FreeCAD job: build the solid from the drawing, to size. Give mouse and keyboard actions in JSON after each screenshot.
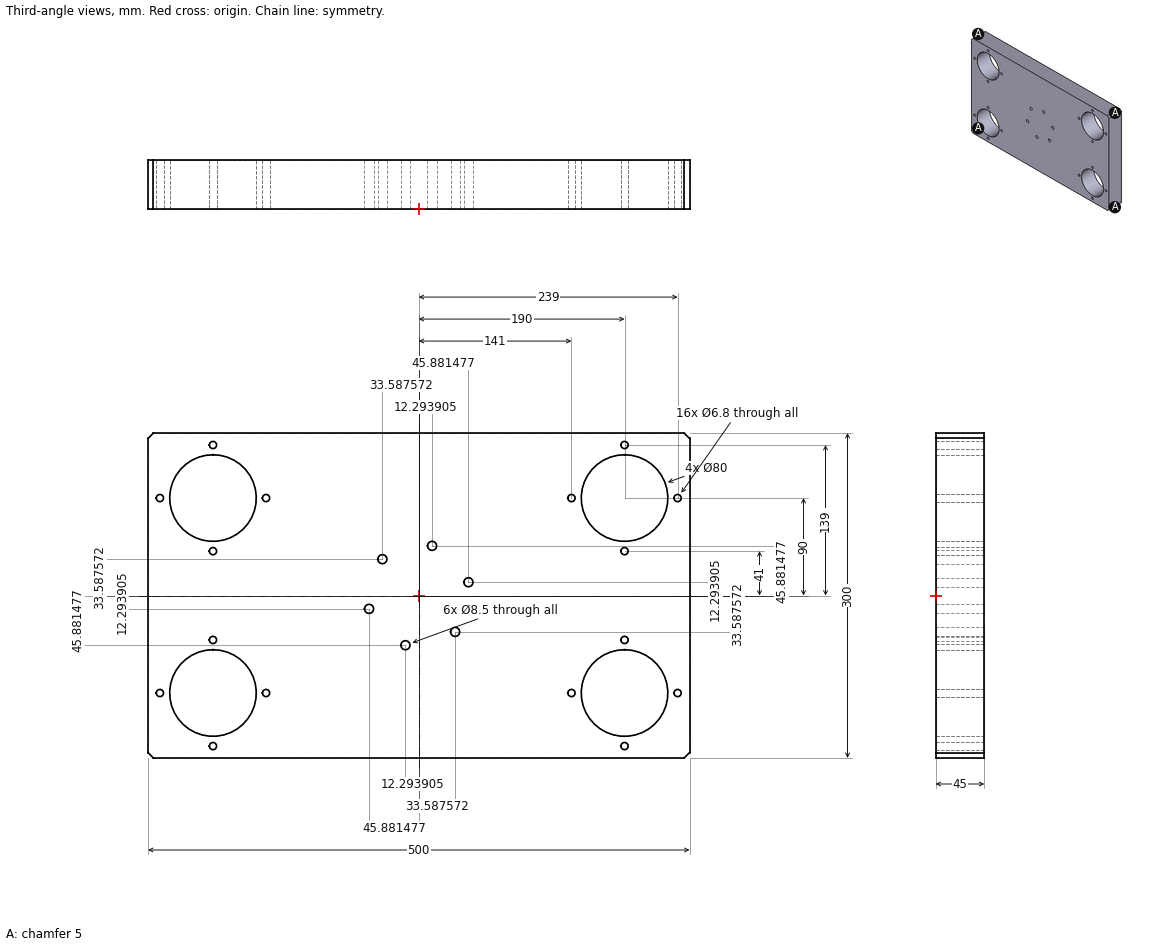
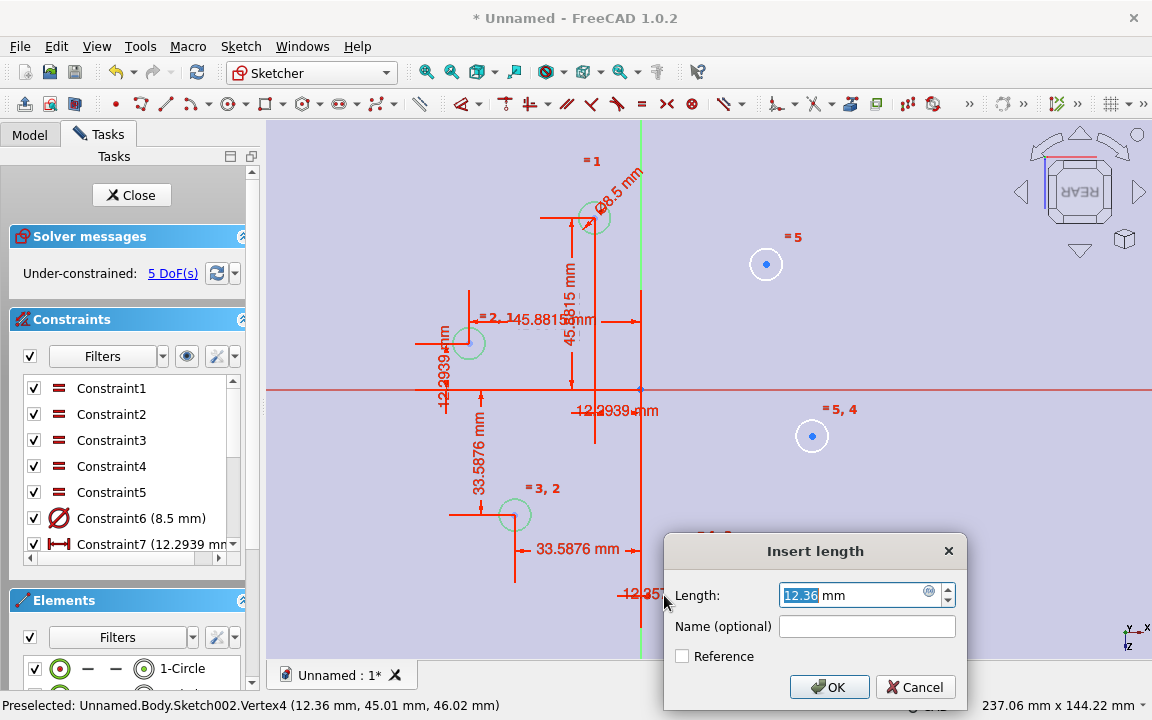
{"action": "type", "text": "12.293905"}
{"action": "key", "text": "Return"}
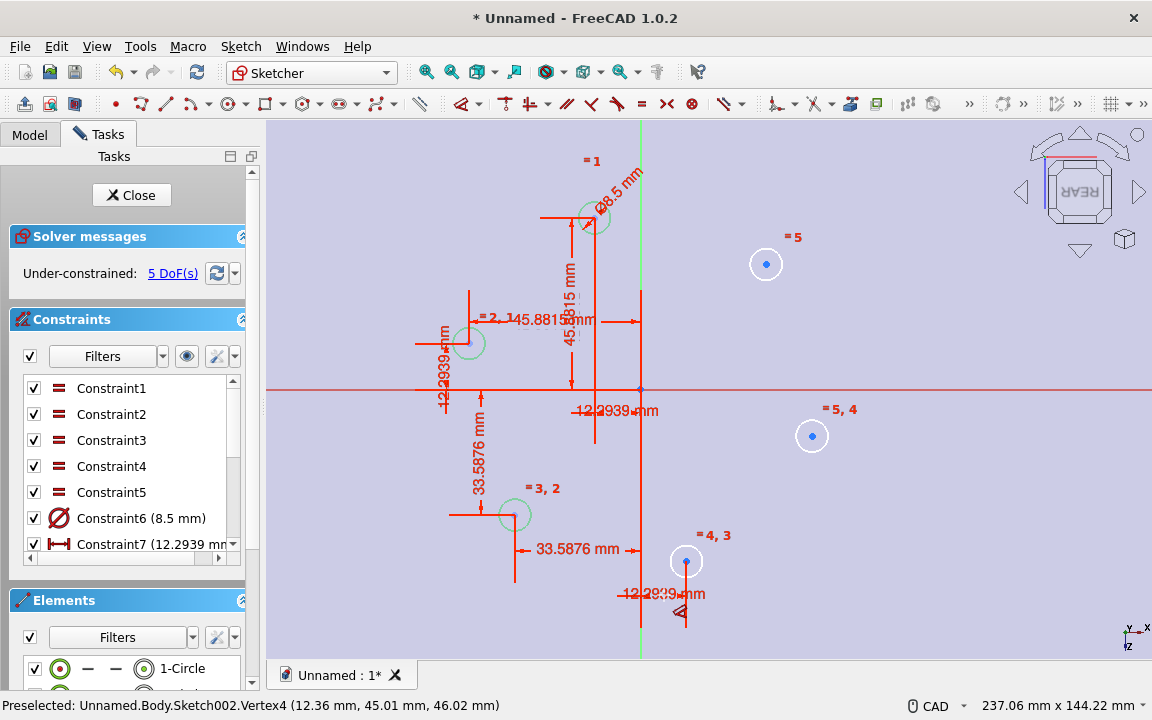
{"action": "left_click", "coordinate": [686, 561]}
{"action": "left_click", "coordinate": [720, 475]}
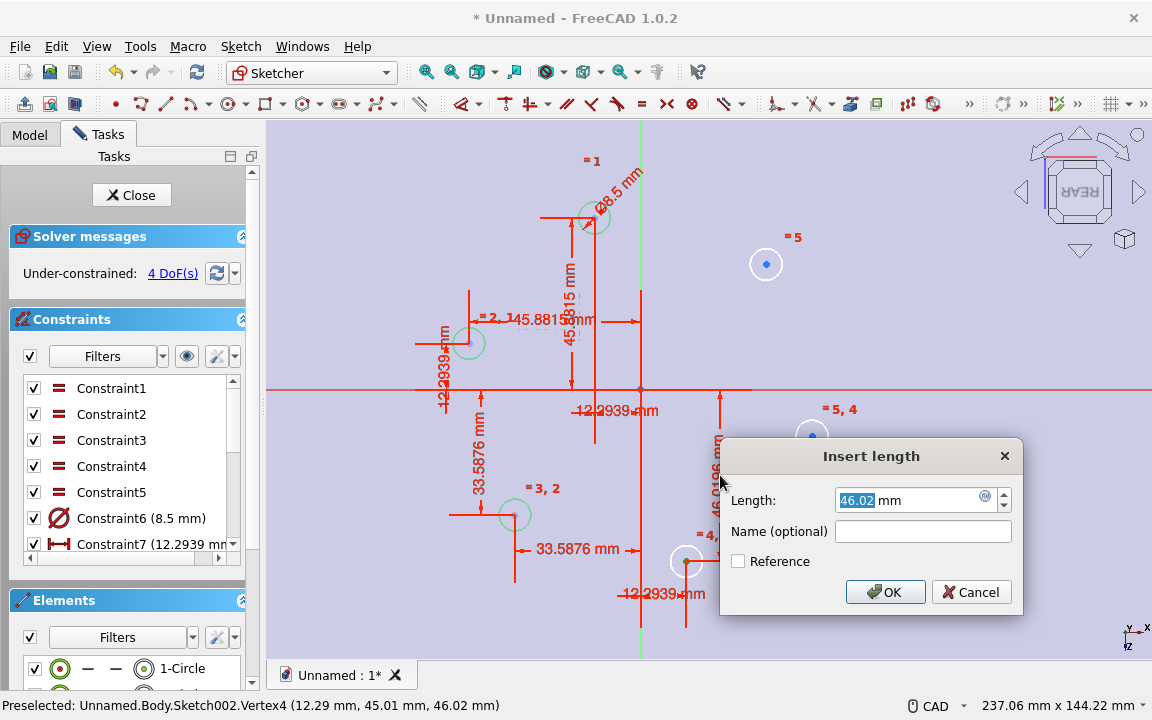
{"action": "type", "text": "45.881477"}
{"action": "key", "text": "Return"}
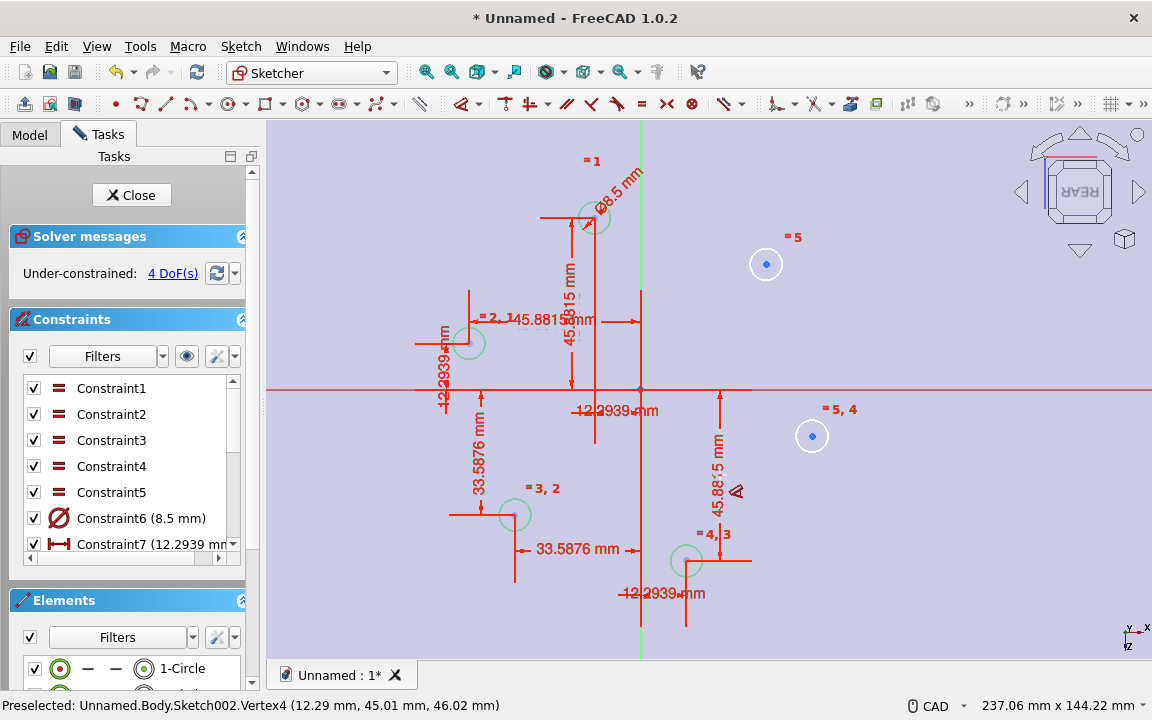
{"action": "left_click", "coordinate": [812, 436]}
{"action": "left_click", "coordinate": [726, 355]}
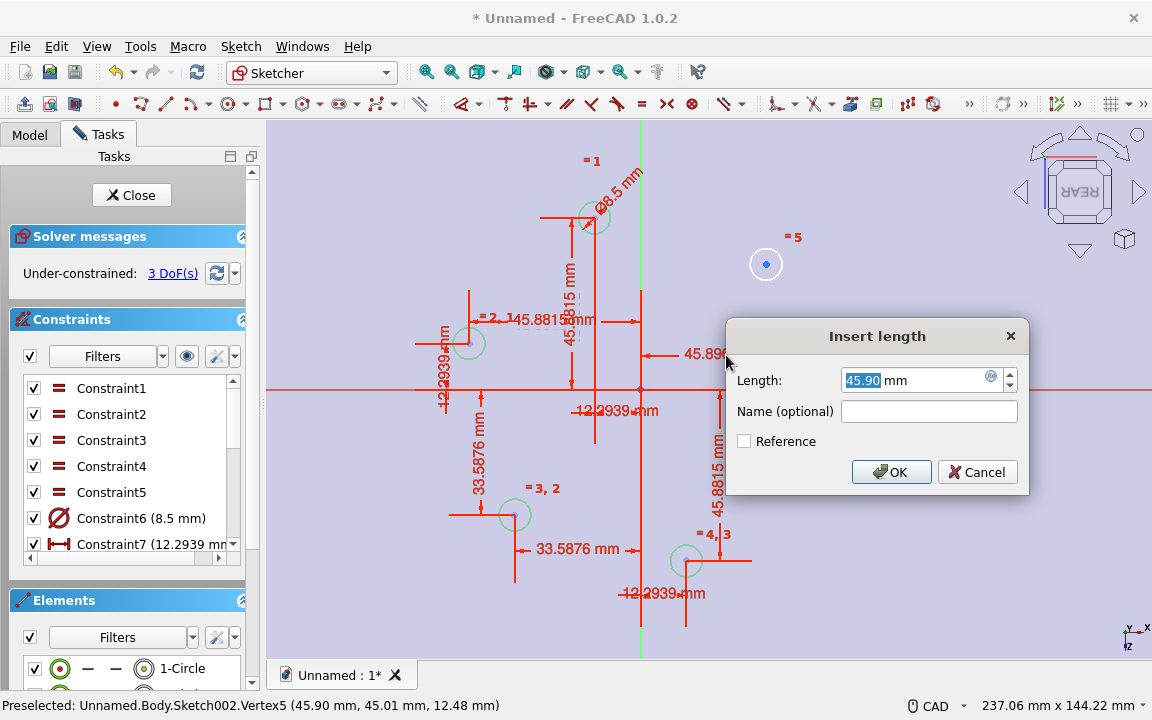
{"action": "type", "text": "45.881477"}
{"action": "key", "text": "Return"}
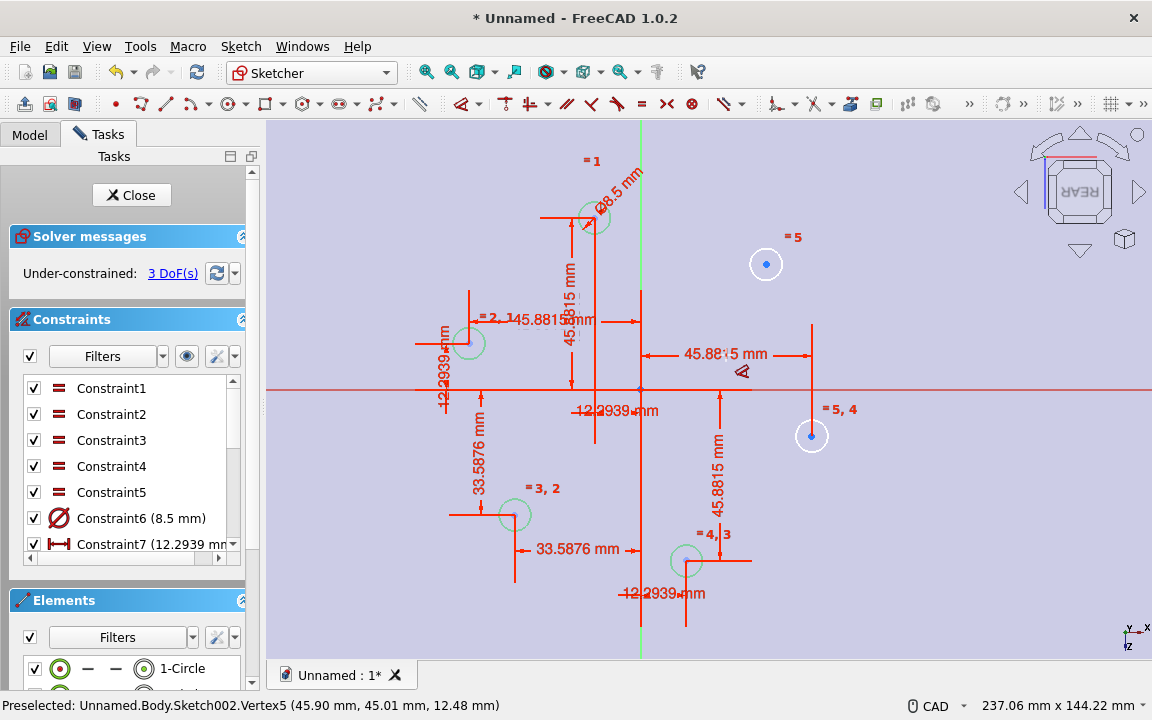
{"action": "left_click", "coordinate": [812, 436]}
{"action": "left_click", "coordinate": [846, 413]}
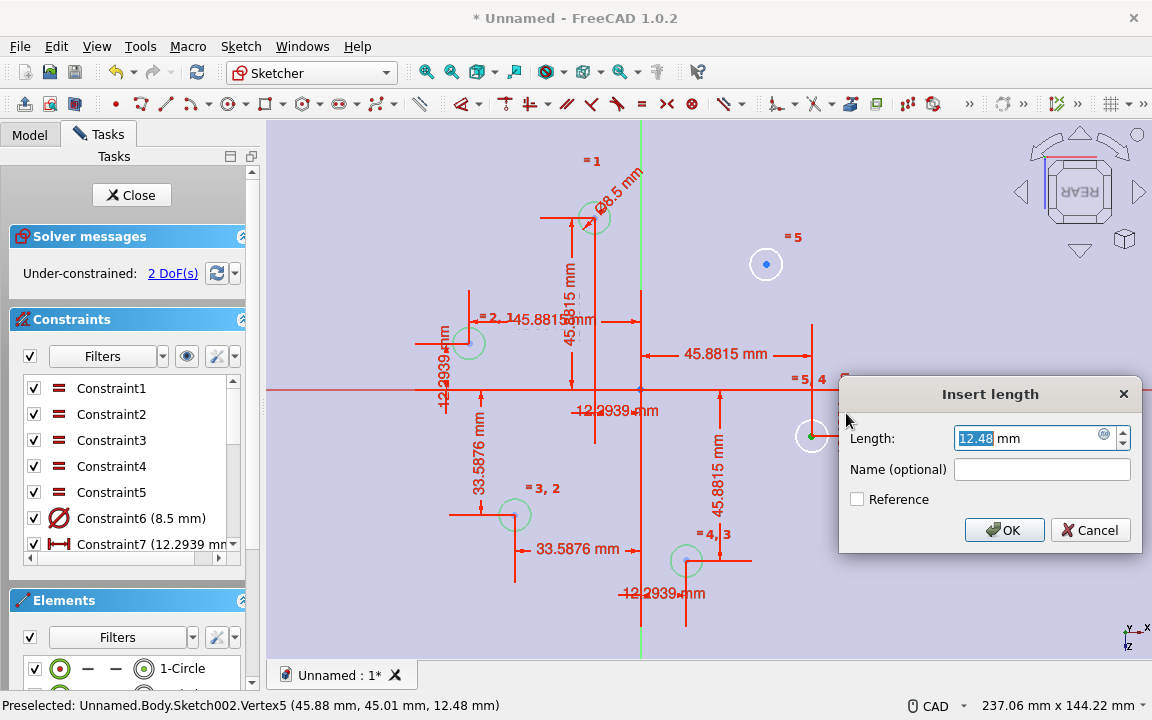
{"action": "type", "text": "12.293905"}
{"action": "key", "text": "Return"}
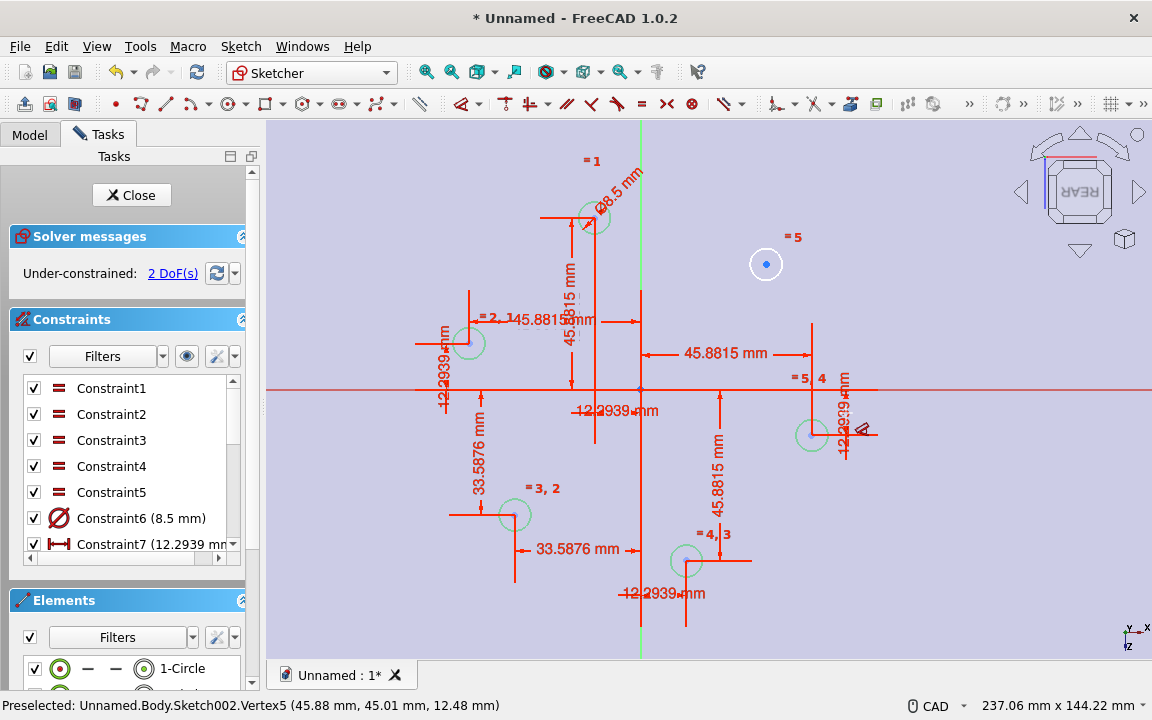
{"action": "left_click", "coordinate": [766, 264]}
{"action": "left_click", "coordinate": [703, 230]}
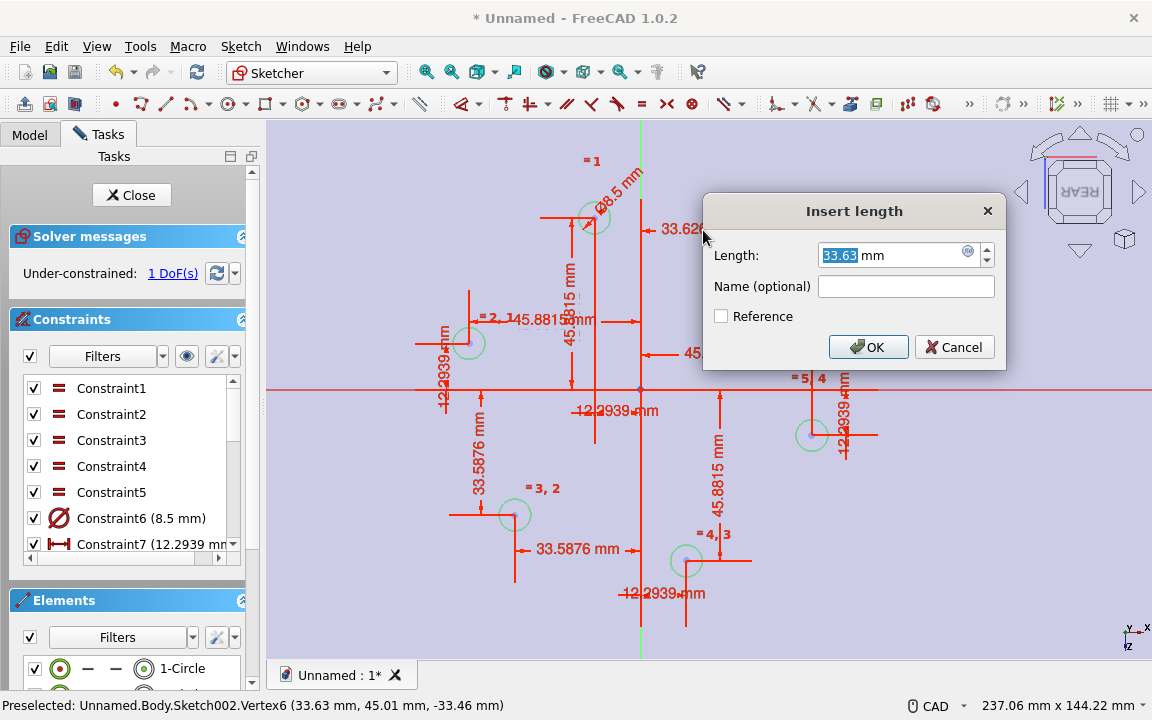
{"action": "type", "text": "33.587572"}
{"action": "key", "text": "Return"}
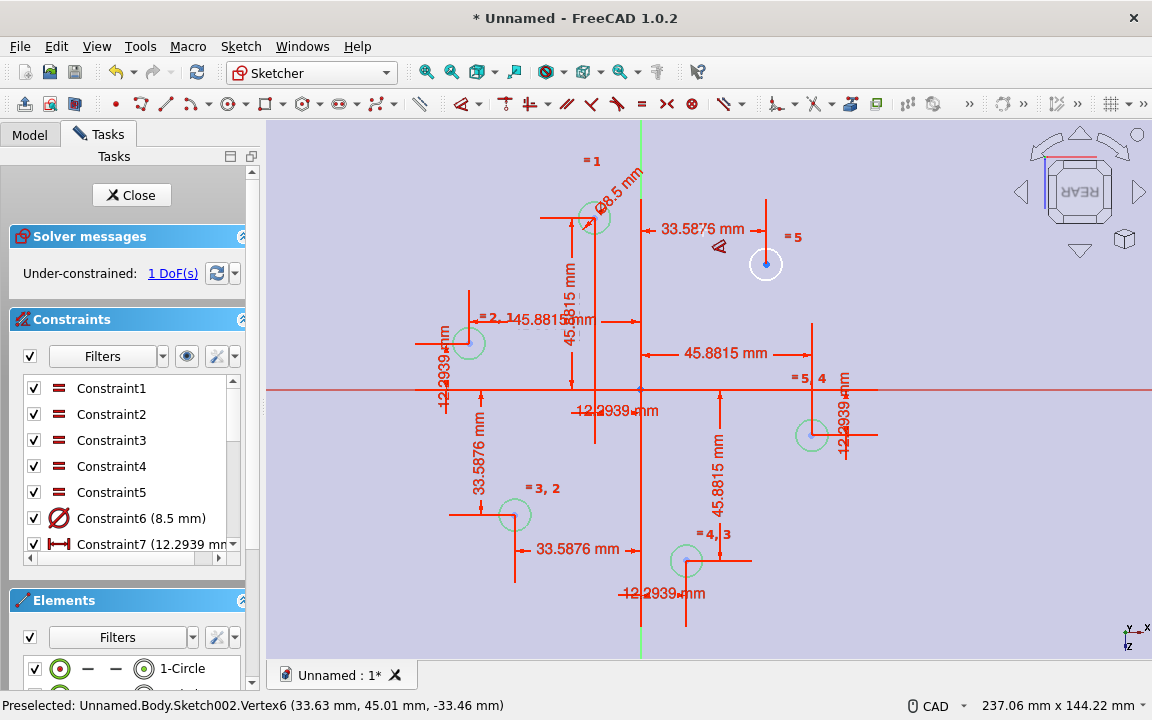
{"action": "left_click", "coordinate": [766, 264]}
{"action": "left_click", "coordinate": [800, 327]}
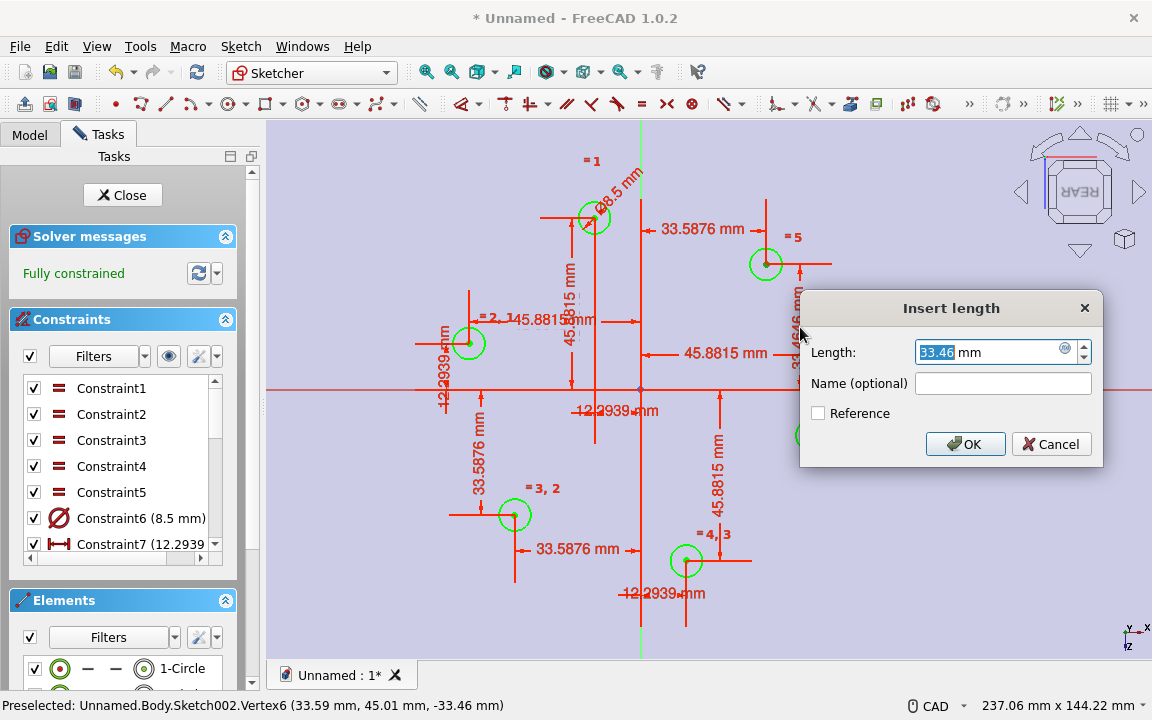
{"action": "type", "text": "33.587572"}
{"action": "key", "text": "Return"}
{"action": "key", "text": "Escape"}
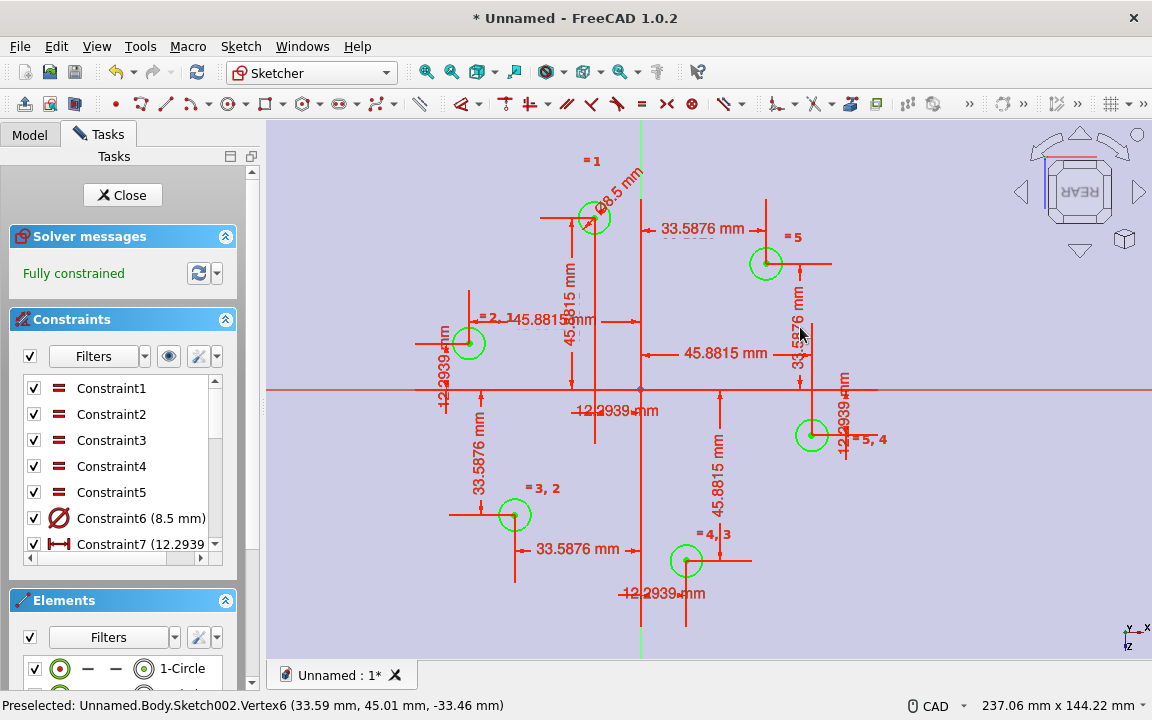
{"action": "left_click", "coordinate": [123, 195]}